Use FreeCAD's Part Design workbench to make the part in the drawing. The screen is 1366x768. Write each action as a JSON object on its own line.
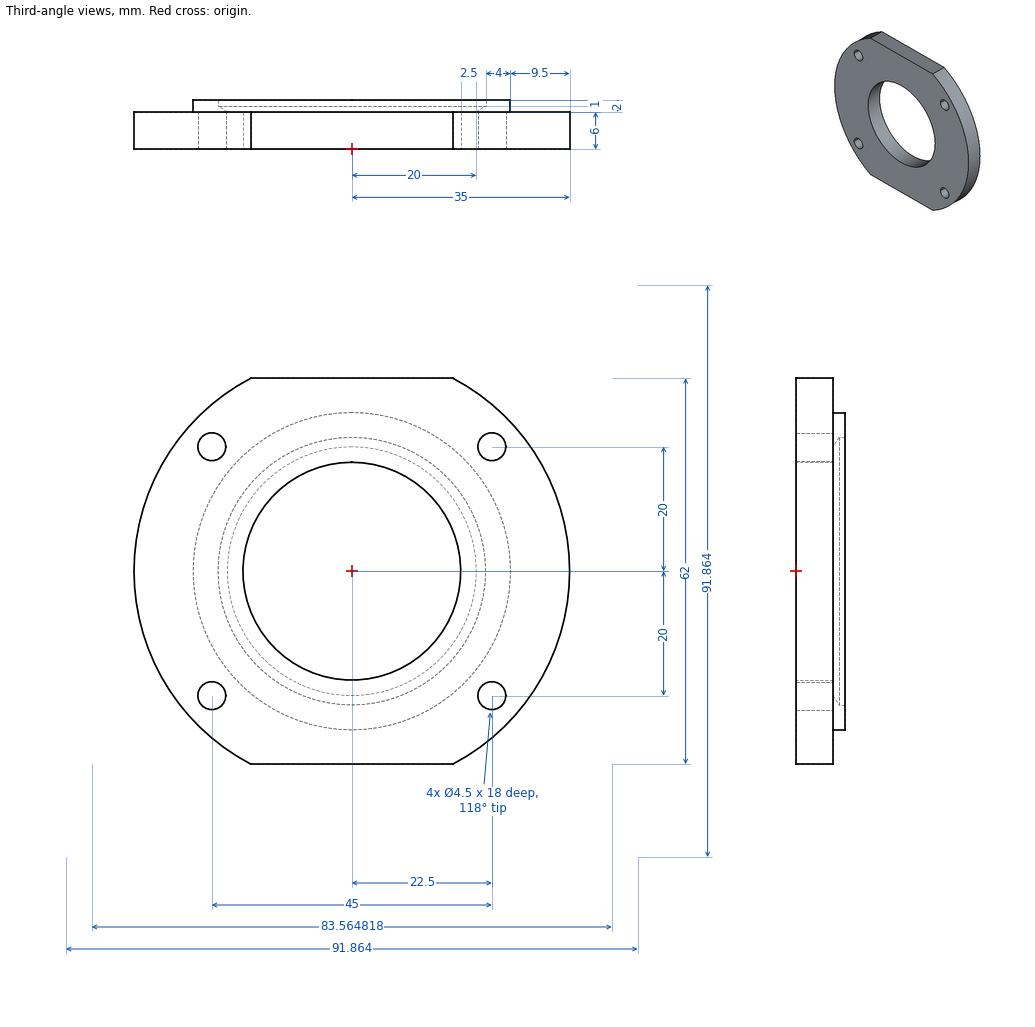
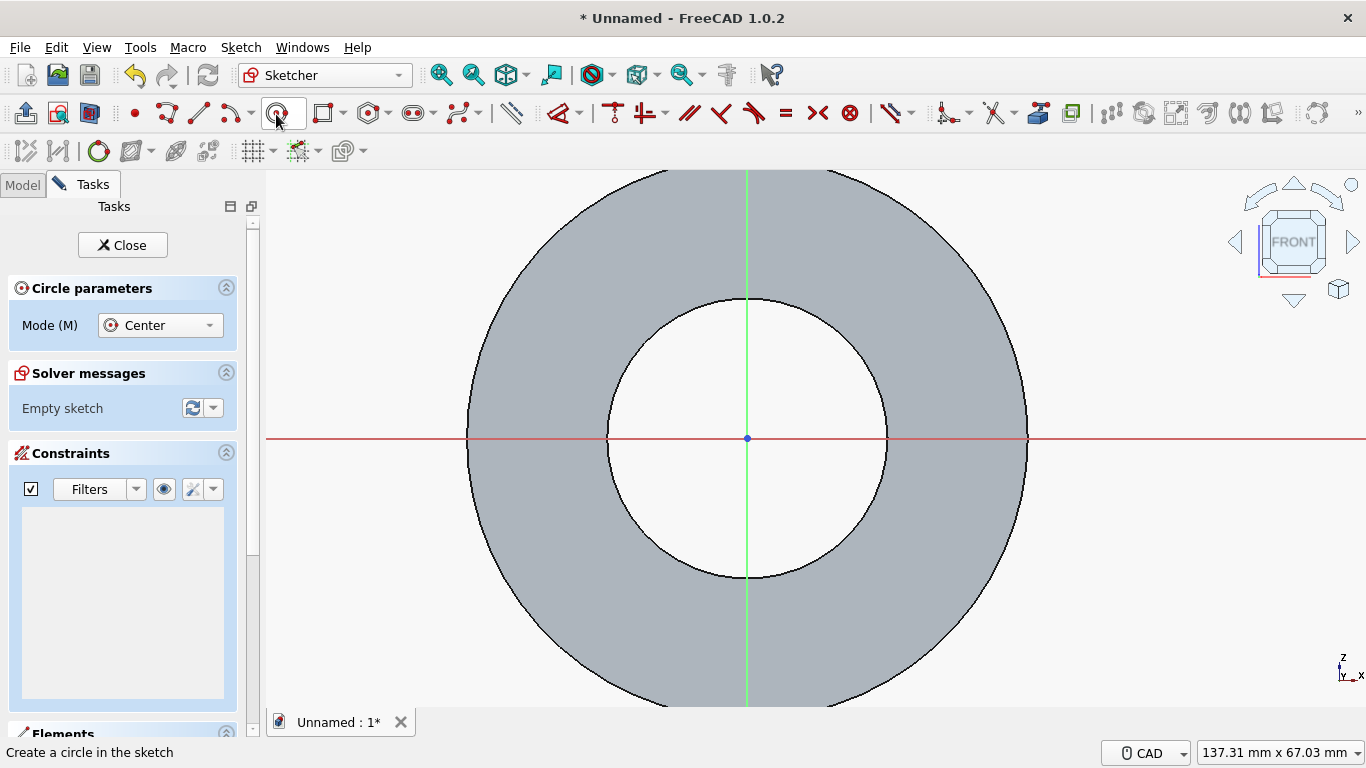
{"action": "scroll", "coordinate": [928, 599], "scroll_direction": "up", "scroll_amount": 2}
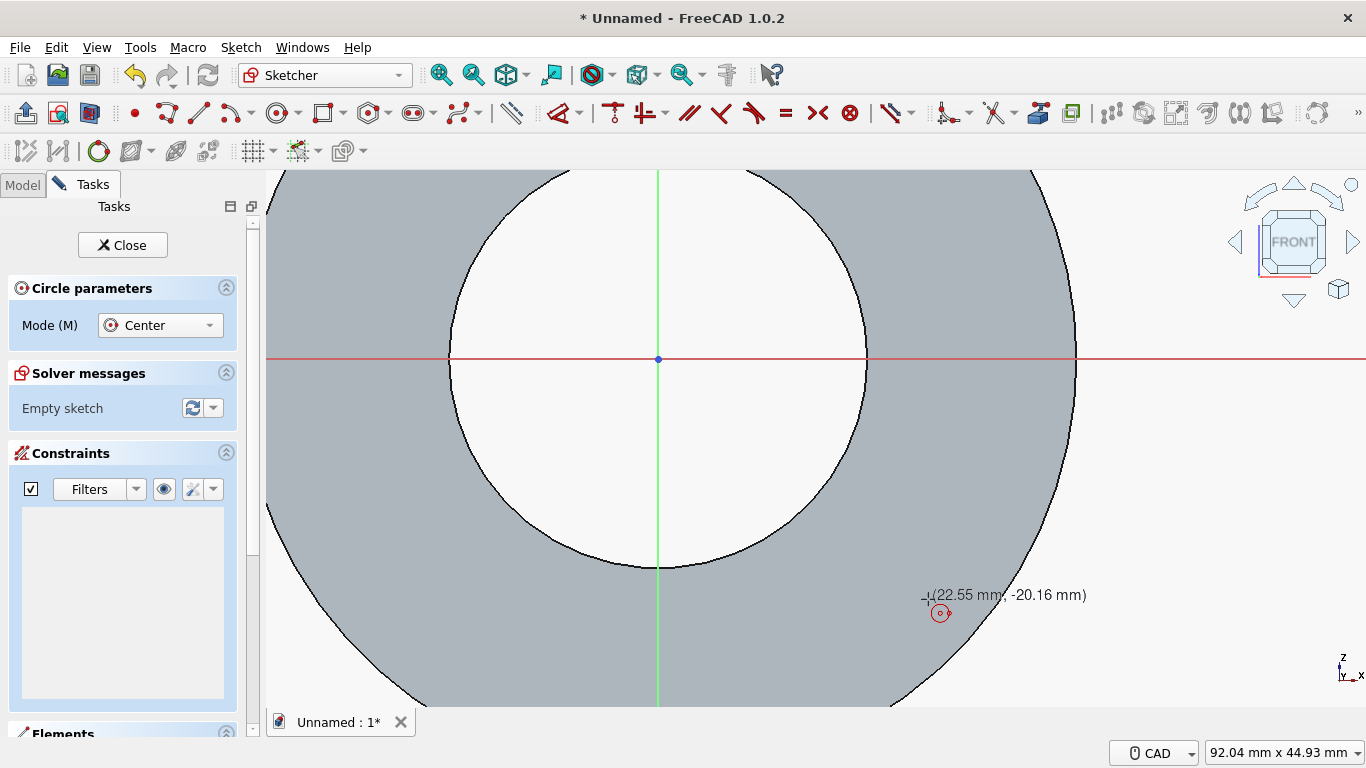
{"action": "left_click", "coordinate": [927, 598]}
{"action": "left_click", "coordinate": [946, 579]}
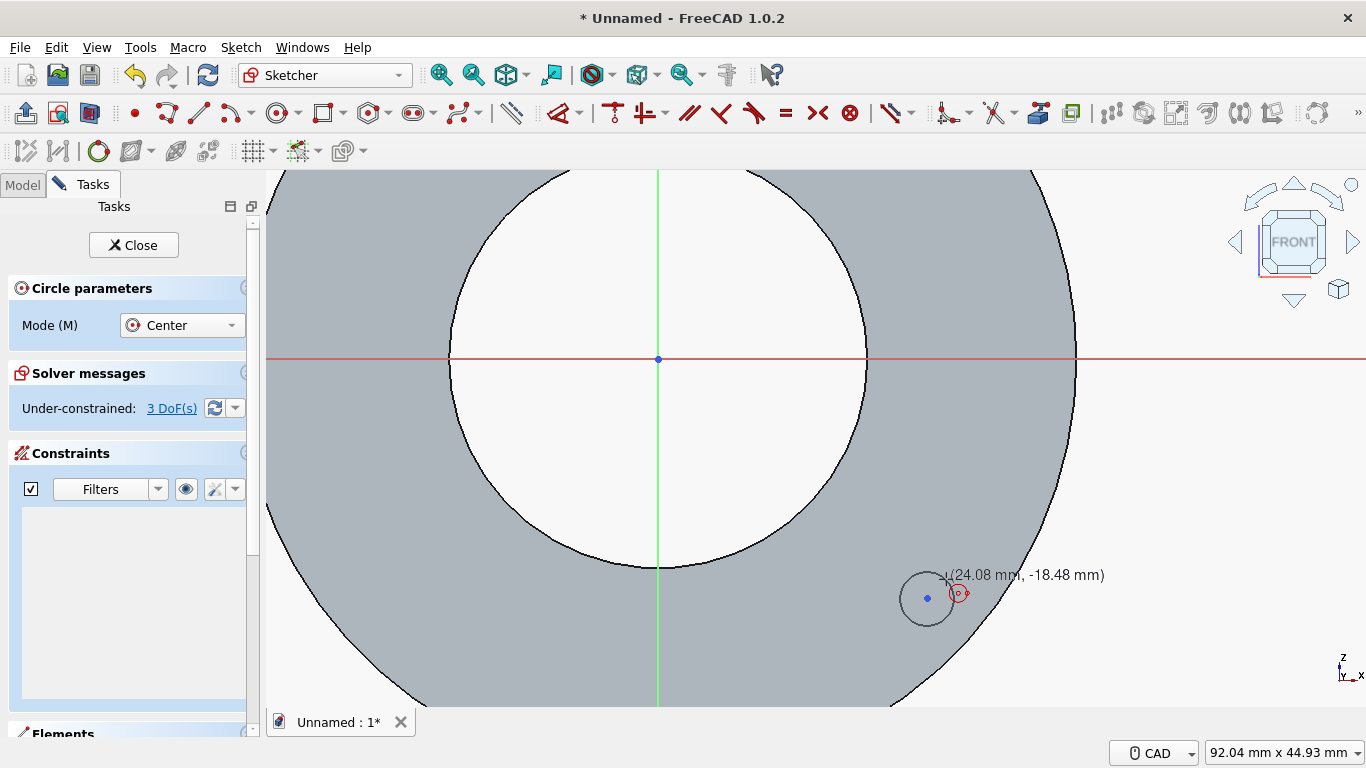
{"action": "scroll", "coordinate": [929, 600], "scroll_direction": "down", "scroll_amount": 2}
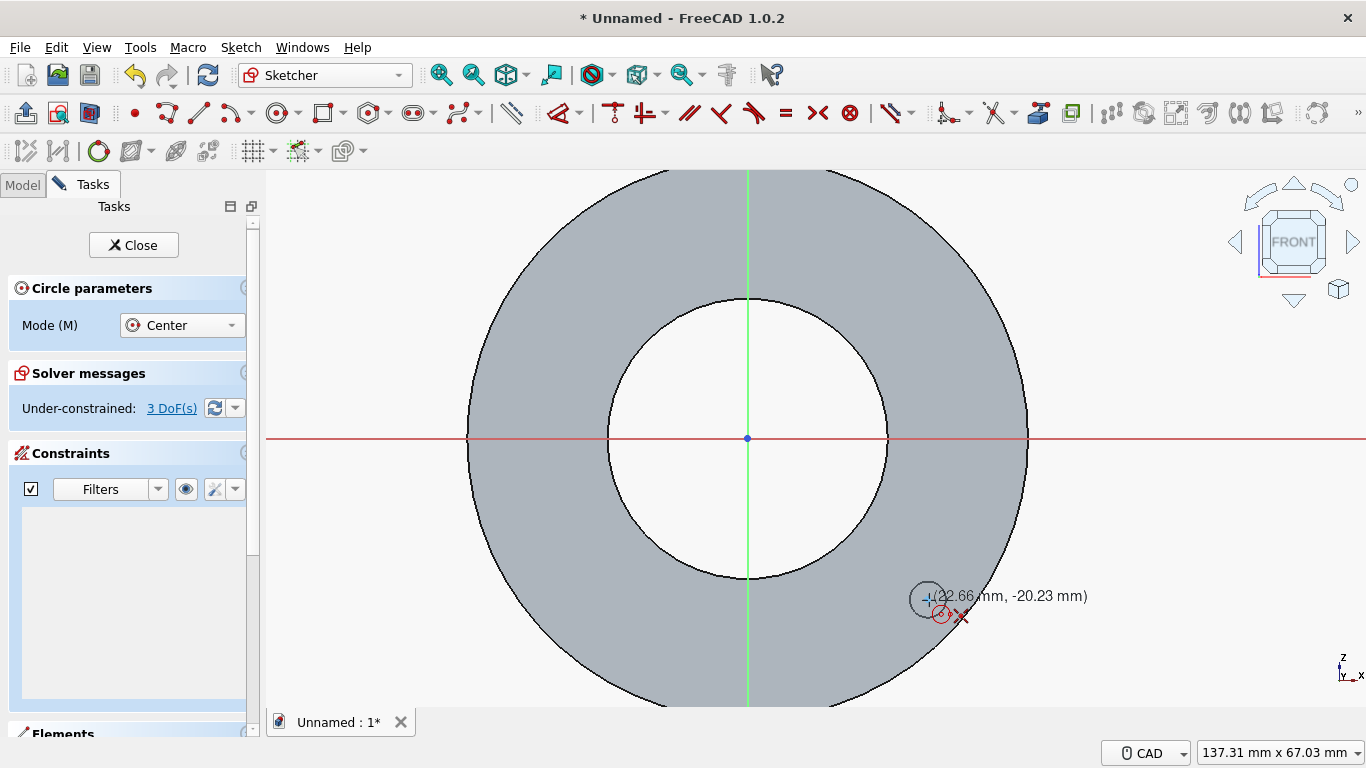
{"action": "scroll", "coordinate": [928, 279], "scroll_direction": "up", "scroll_amount": 2}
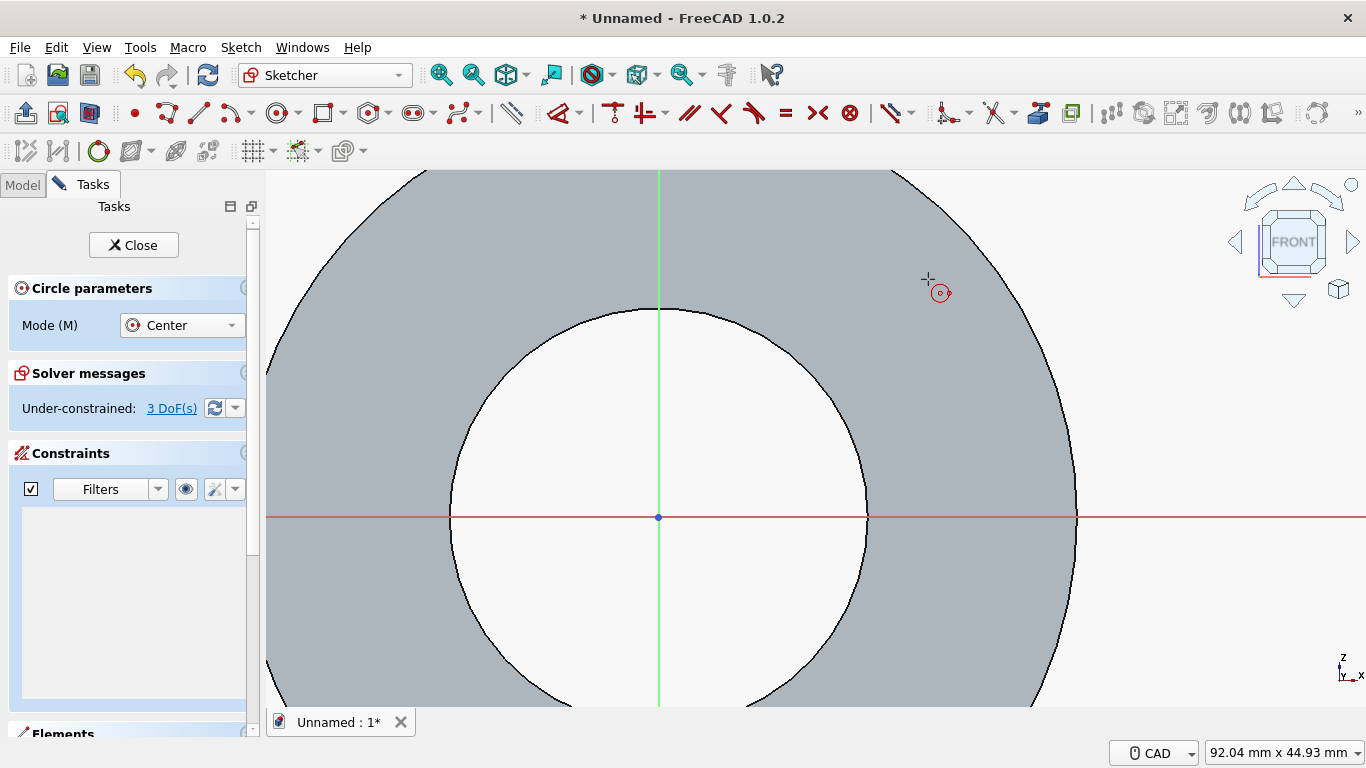
{"action": "left_click", "coordinate": [928, 278]}
{"action": "left_click", "coordinate": [947, 259]}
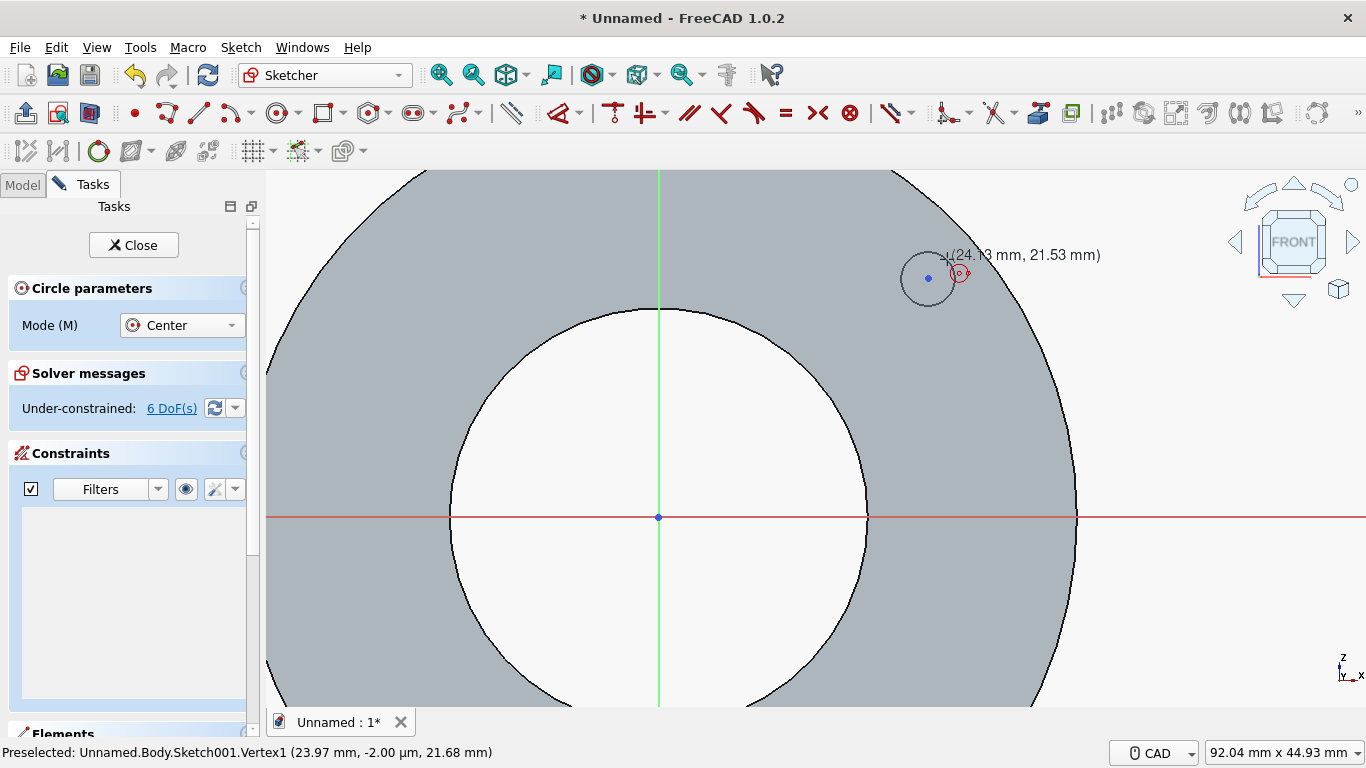
{"action": "scroll", "coordinate": [928, 278], "scroll_direction": "down", "scroll_amount": 2}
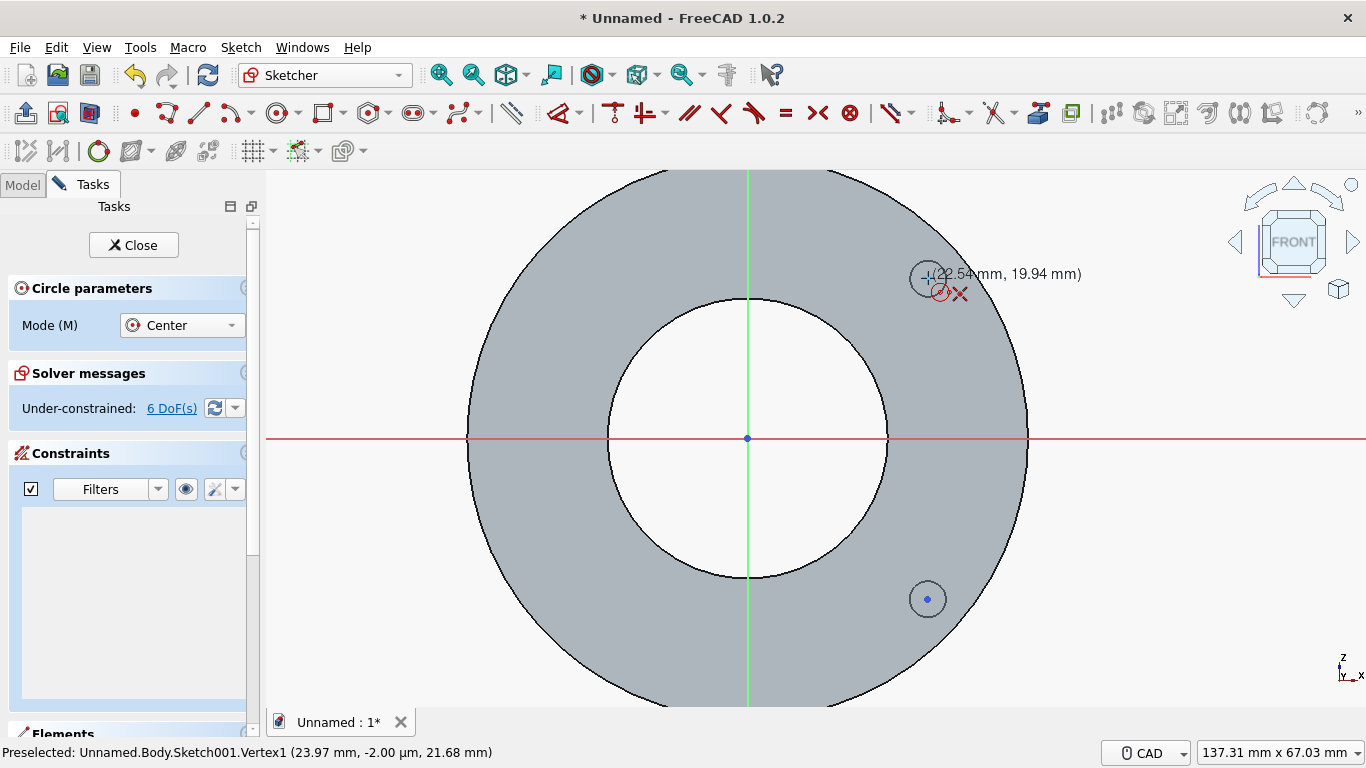
{"action": "scroll", "coordinate": [567, 599], "scroll_direction": "up", "scroll_amount": 2}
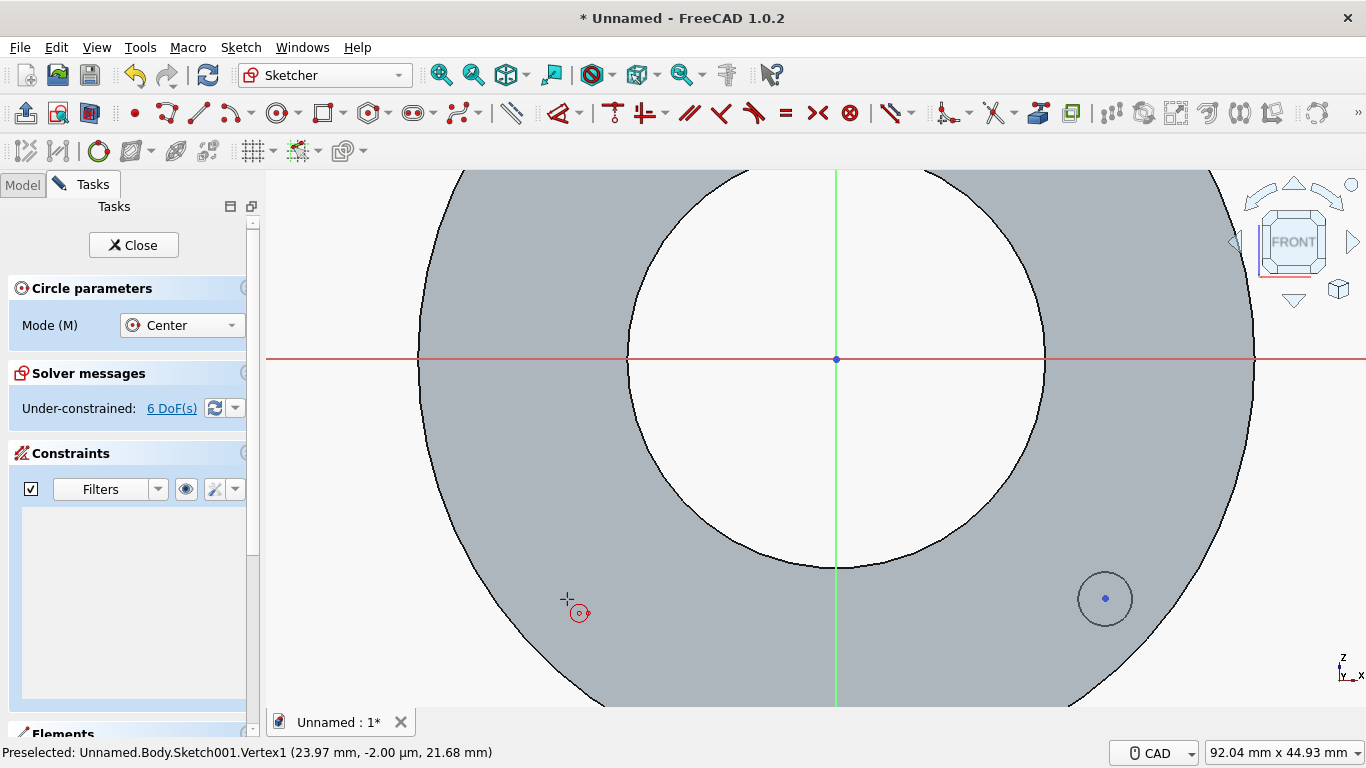
{"action": "left_click", "coordinate": [567, 598]}
{"action": "left_click", "coordinate": [586, 579]}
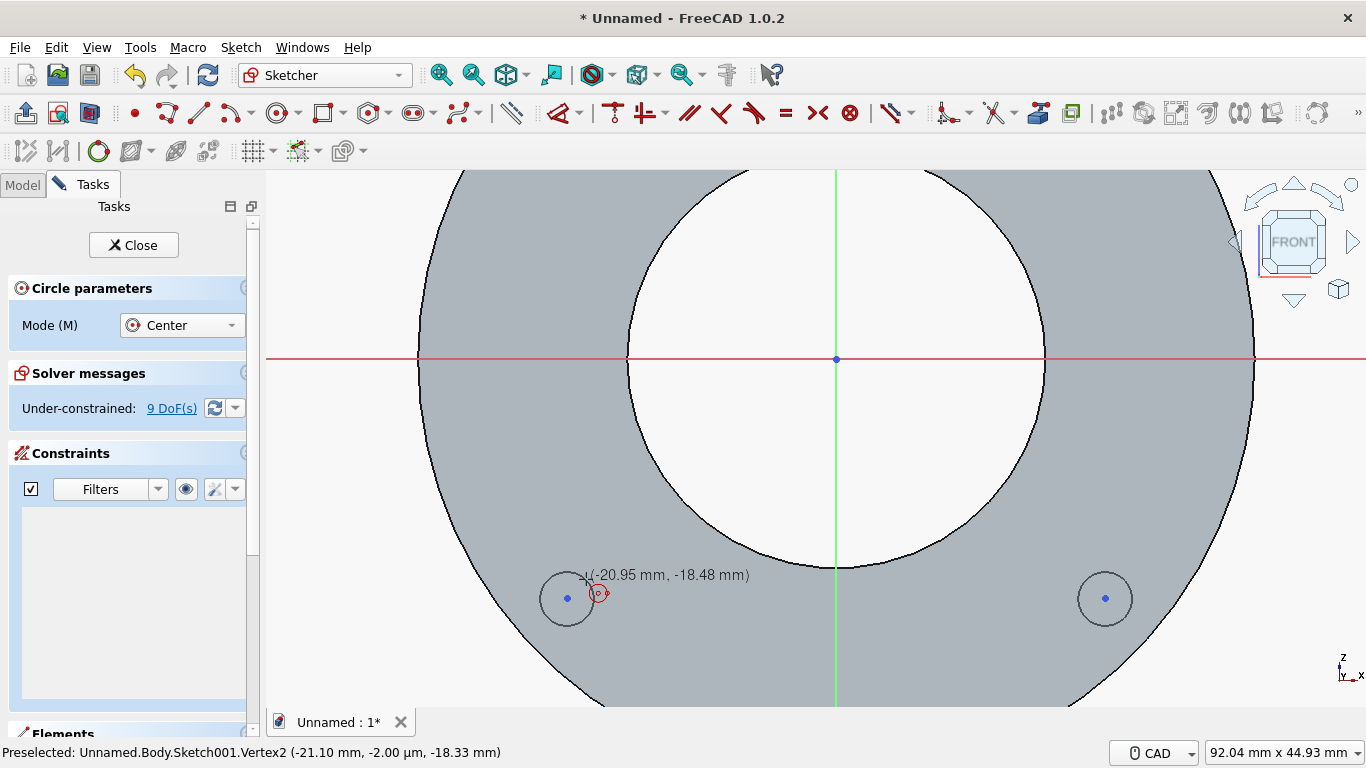
{"action": "scroll", "coordinate": [567, 600], "scroll_direction": "down", "scroll_amount": 2}